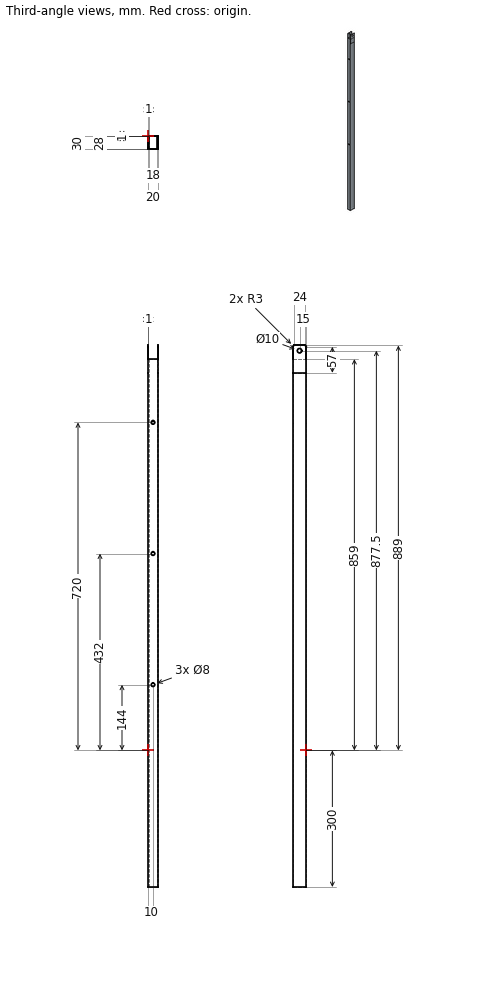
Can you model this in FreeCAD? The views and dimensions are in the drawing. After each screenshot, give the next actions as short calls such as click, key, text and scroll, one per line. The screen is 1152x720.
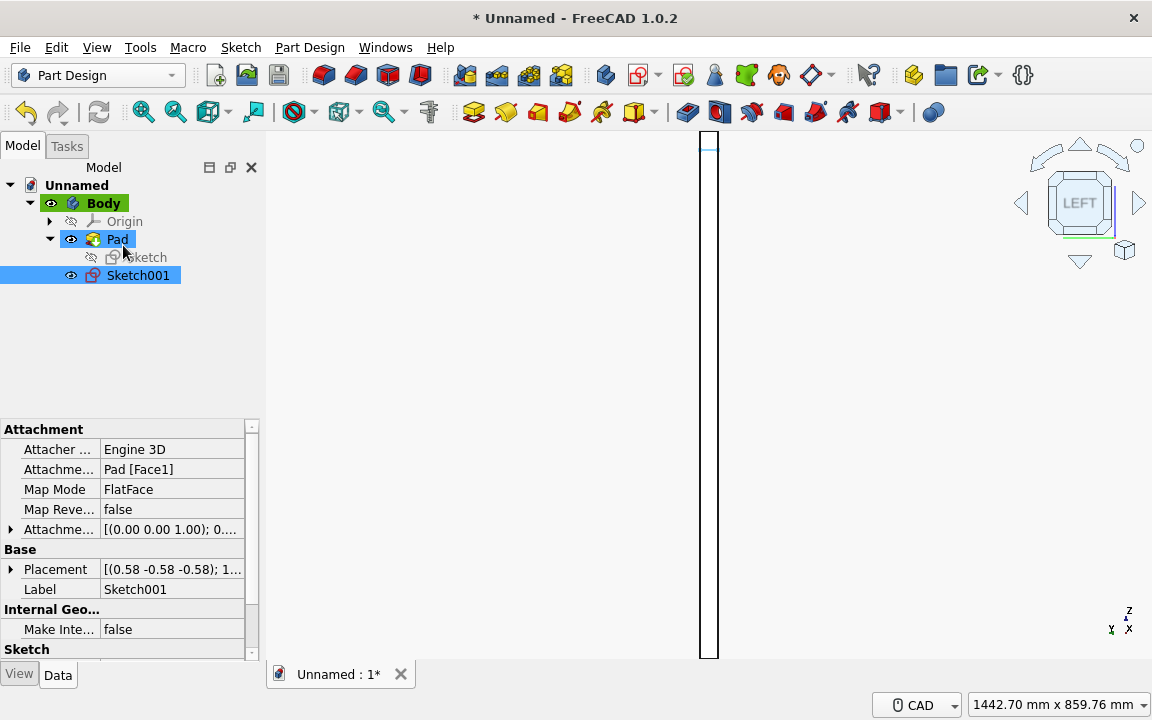
click(474, 112)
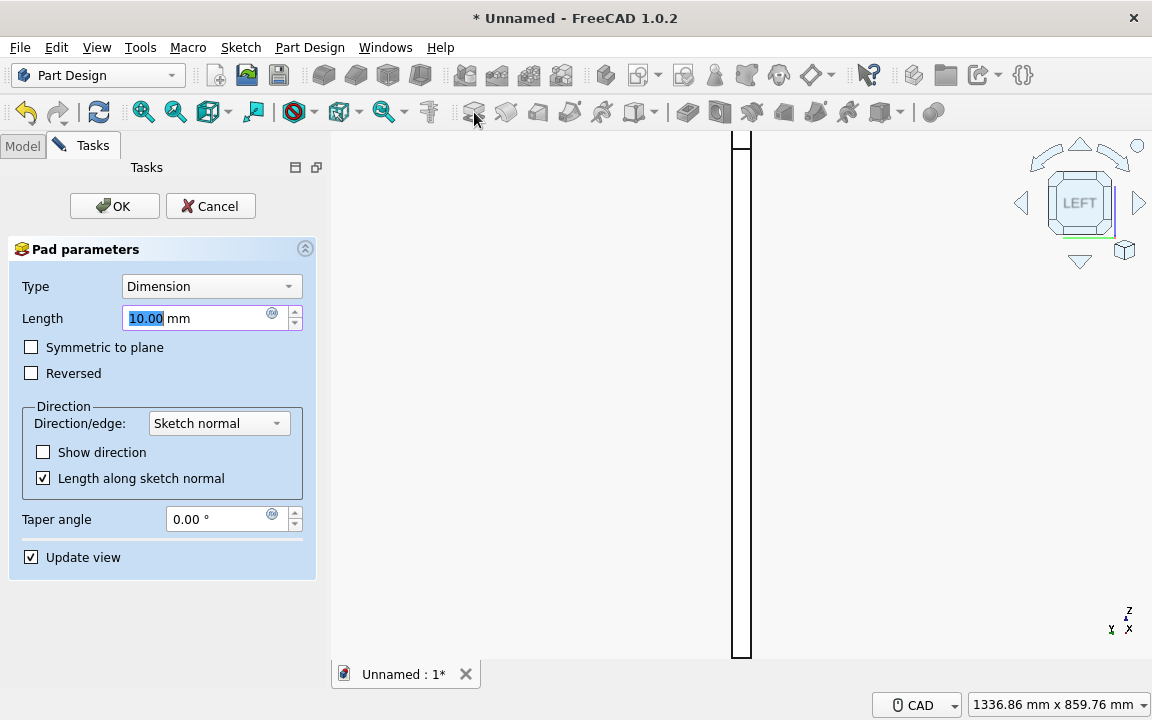
text(1)
key(Tab)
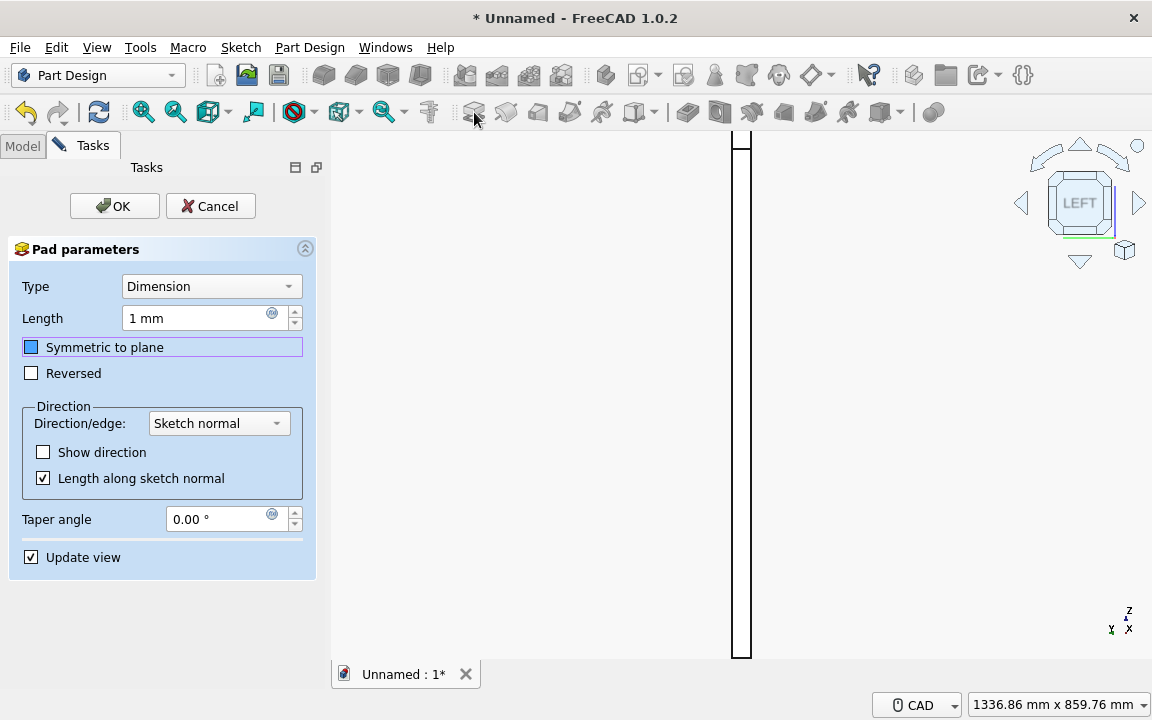
click(115, 206)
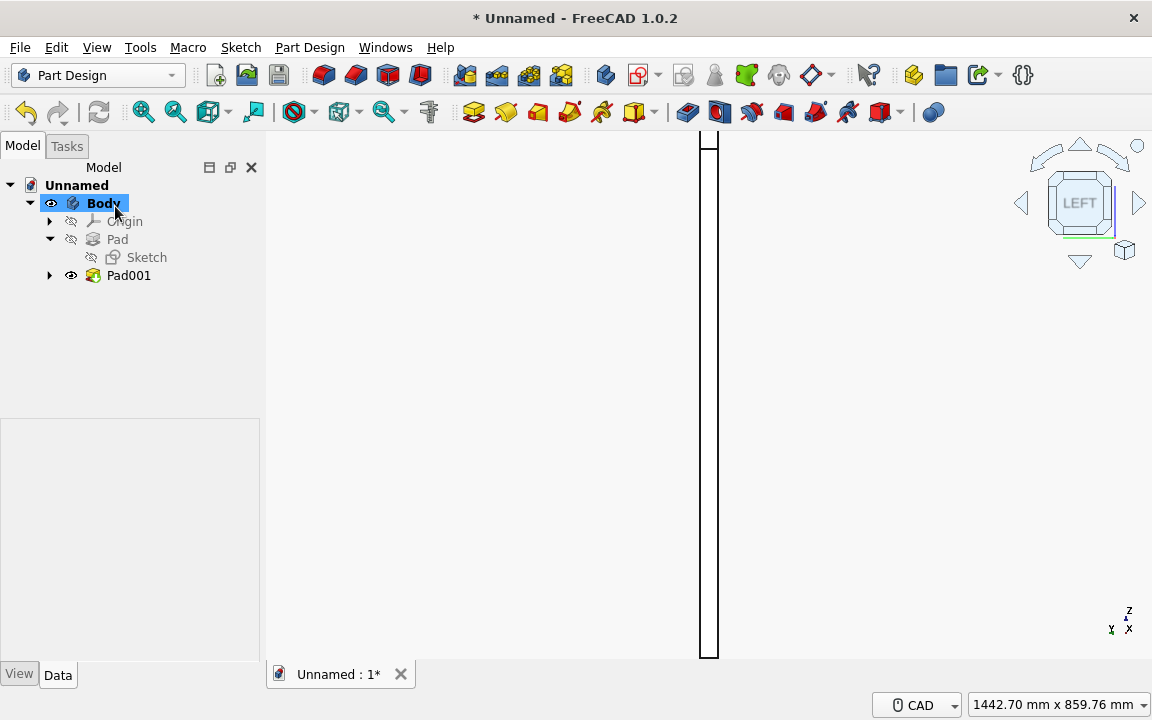
key(v)
key(f)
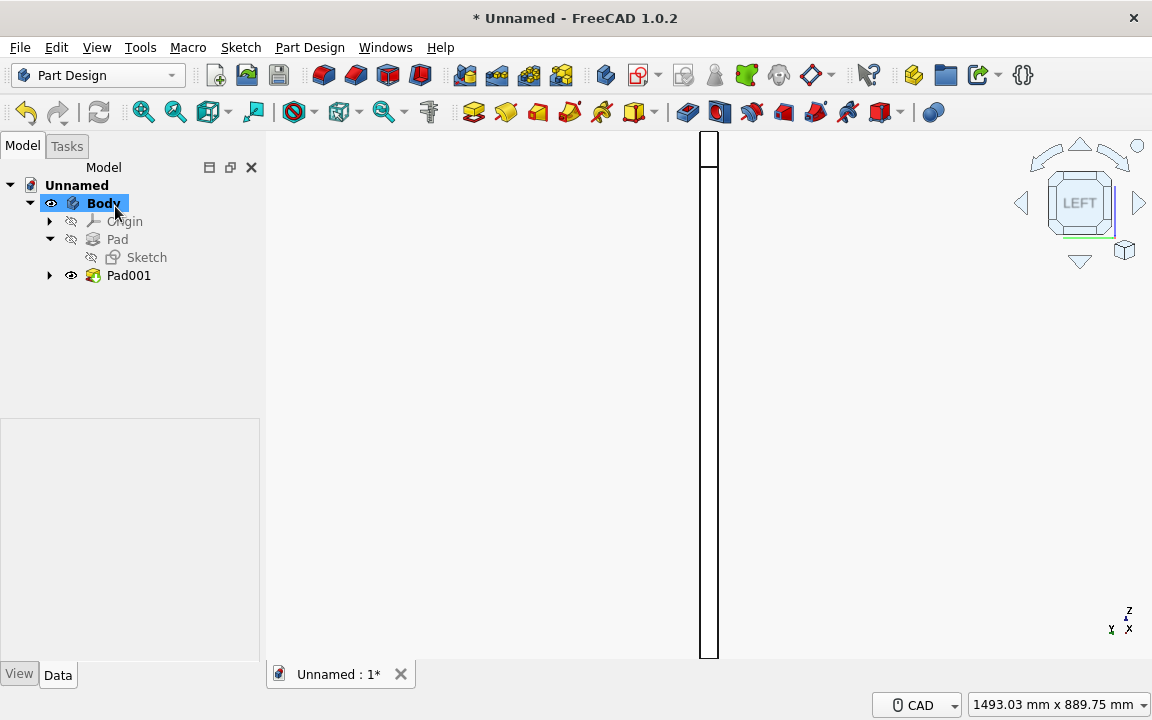
click(50, 221)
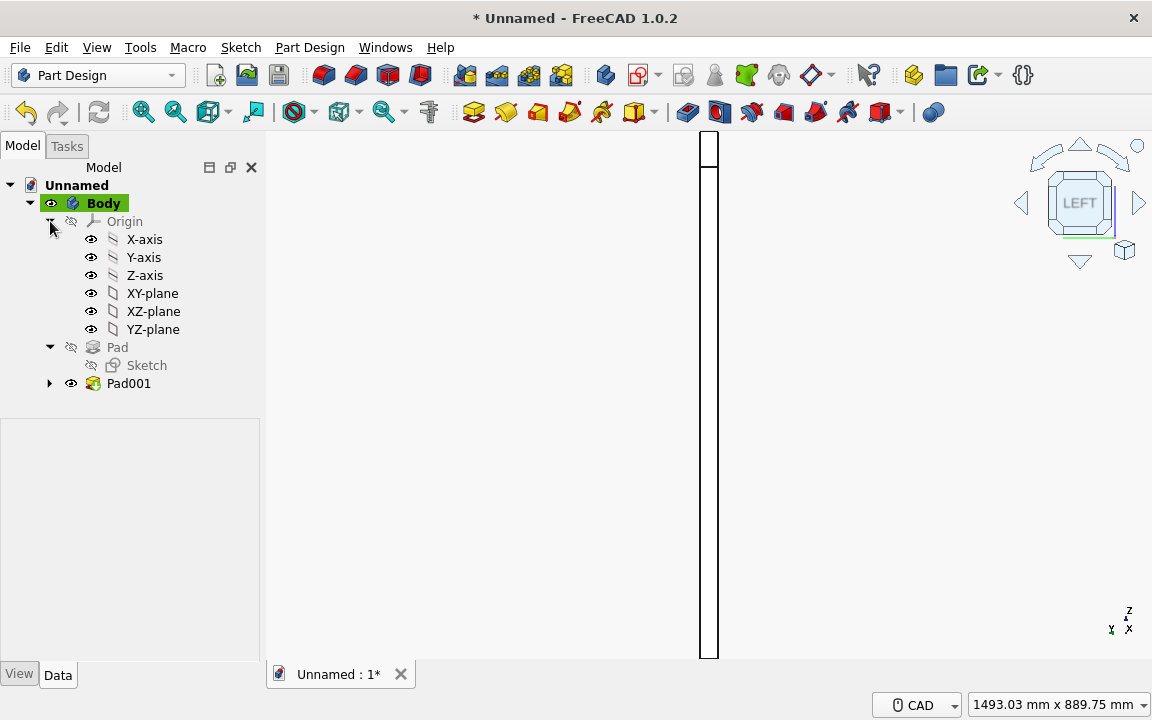
click(136, 329)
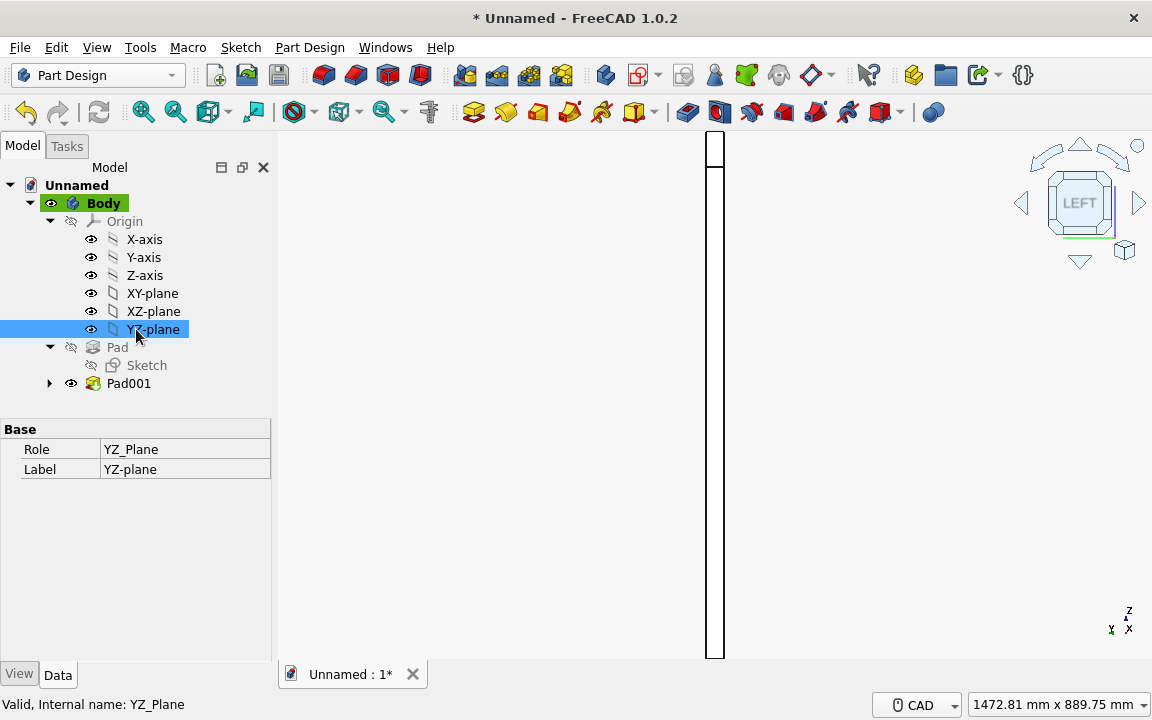
click(812, 76)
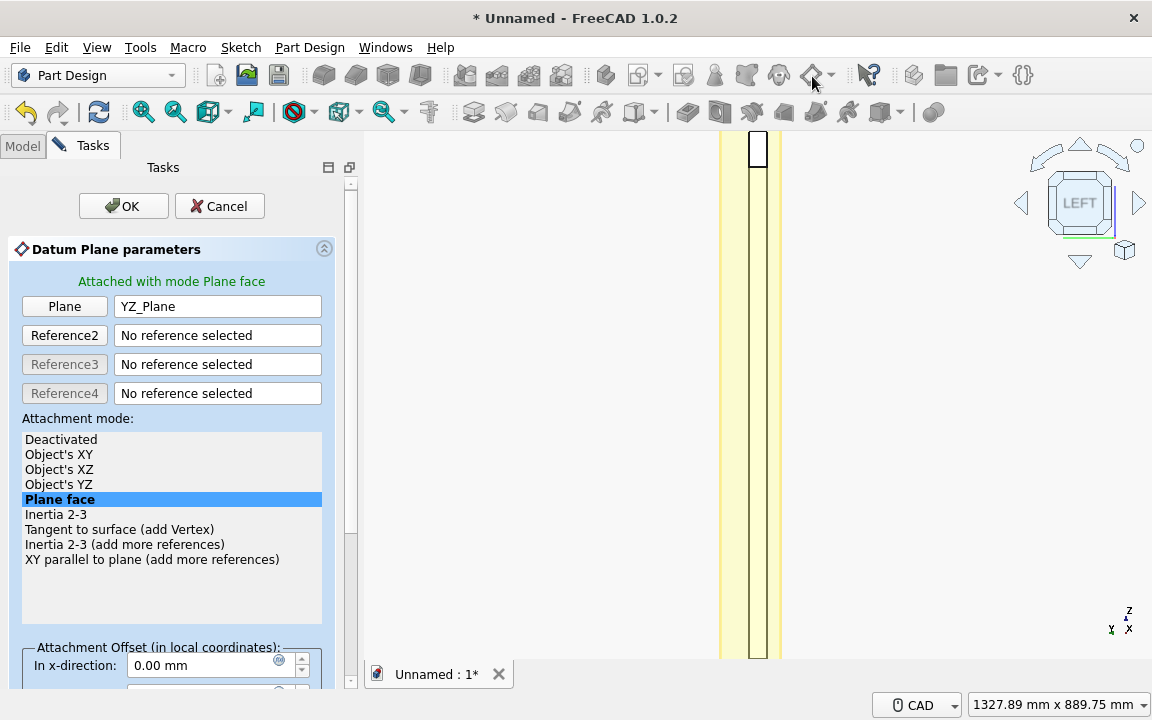
scroll(351, 432, down, 2)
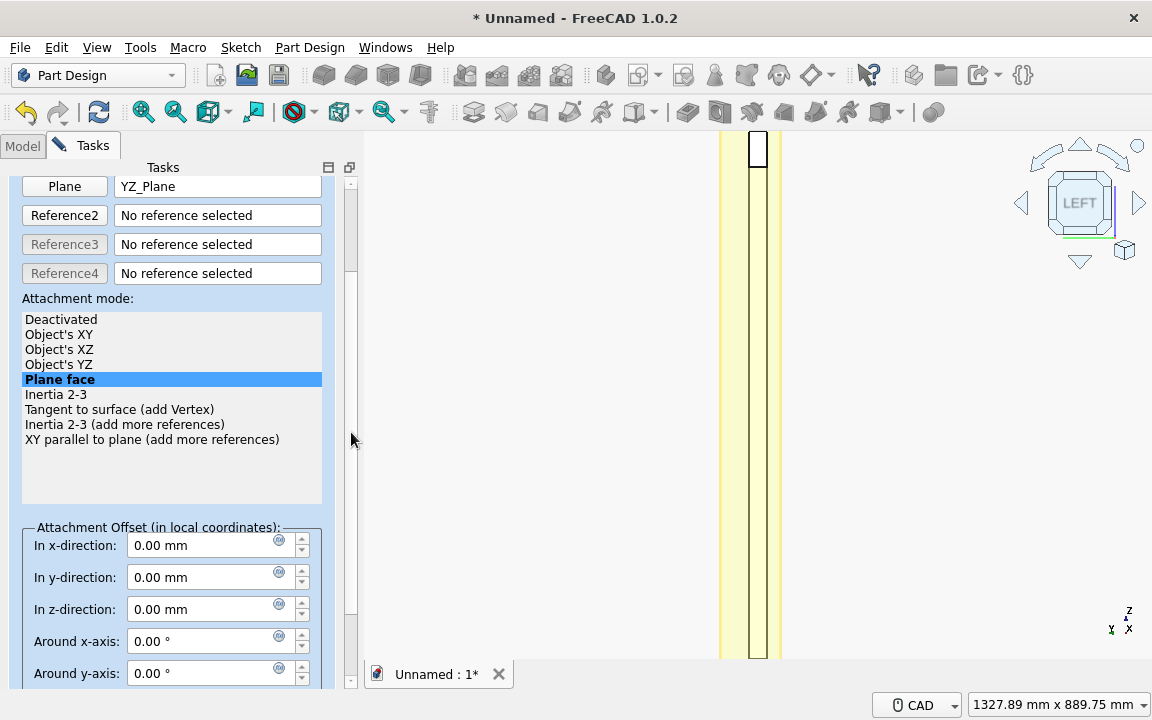
triple_click(210, 609)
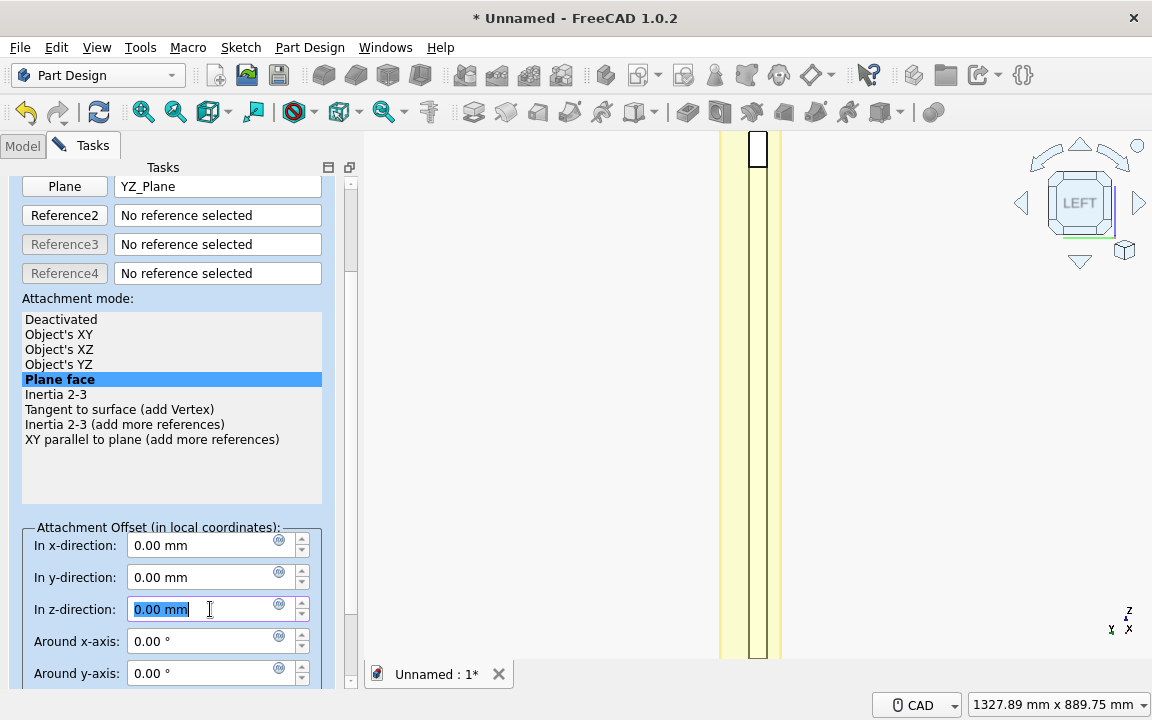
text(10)
key(Tab)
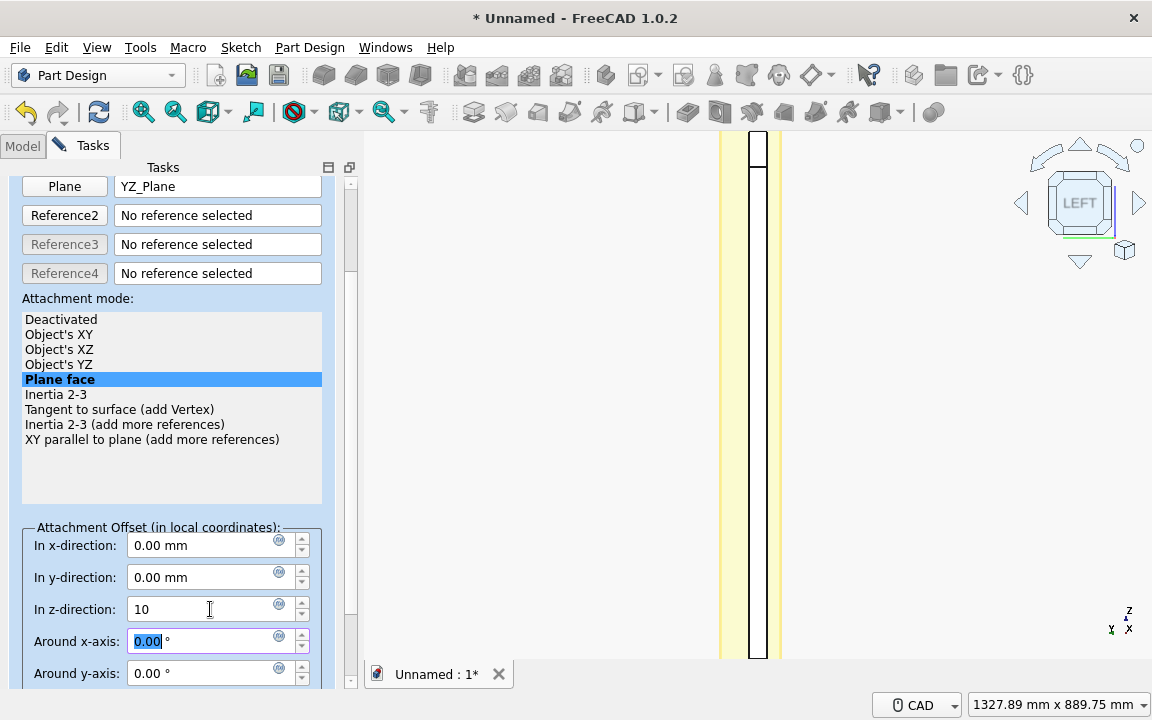
scroll(351, 432, up, 3)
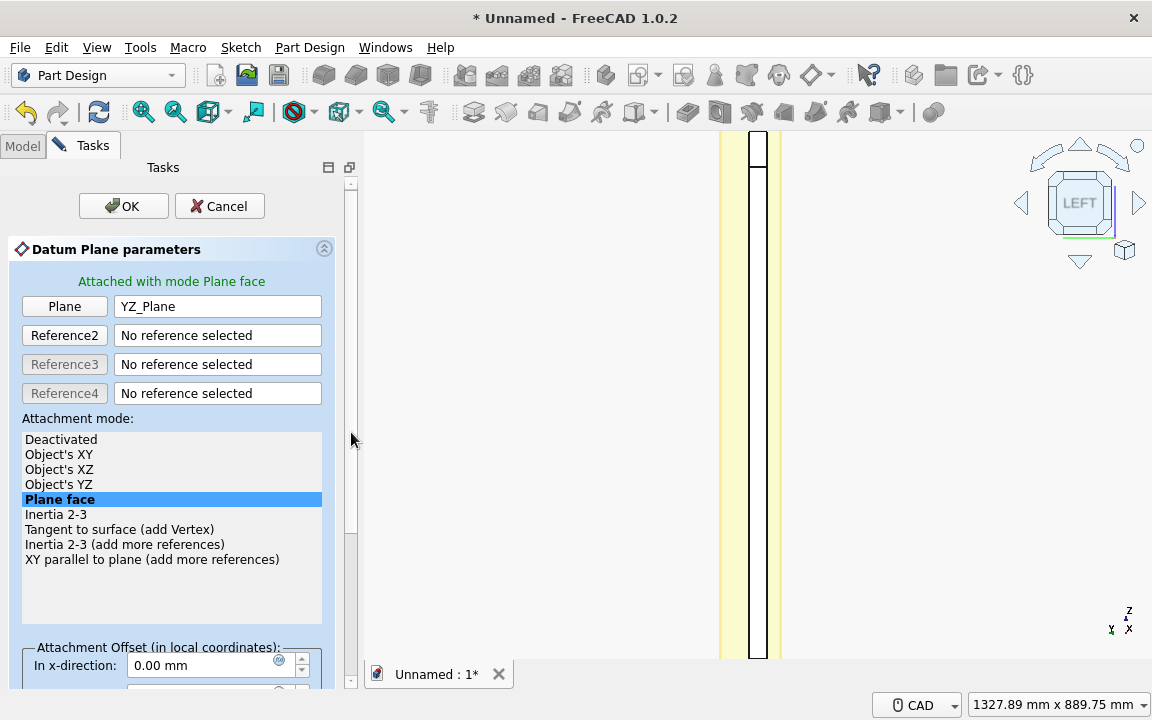
click(124, 206)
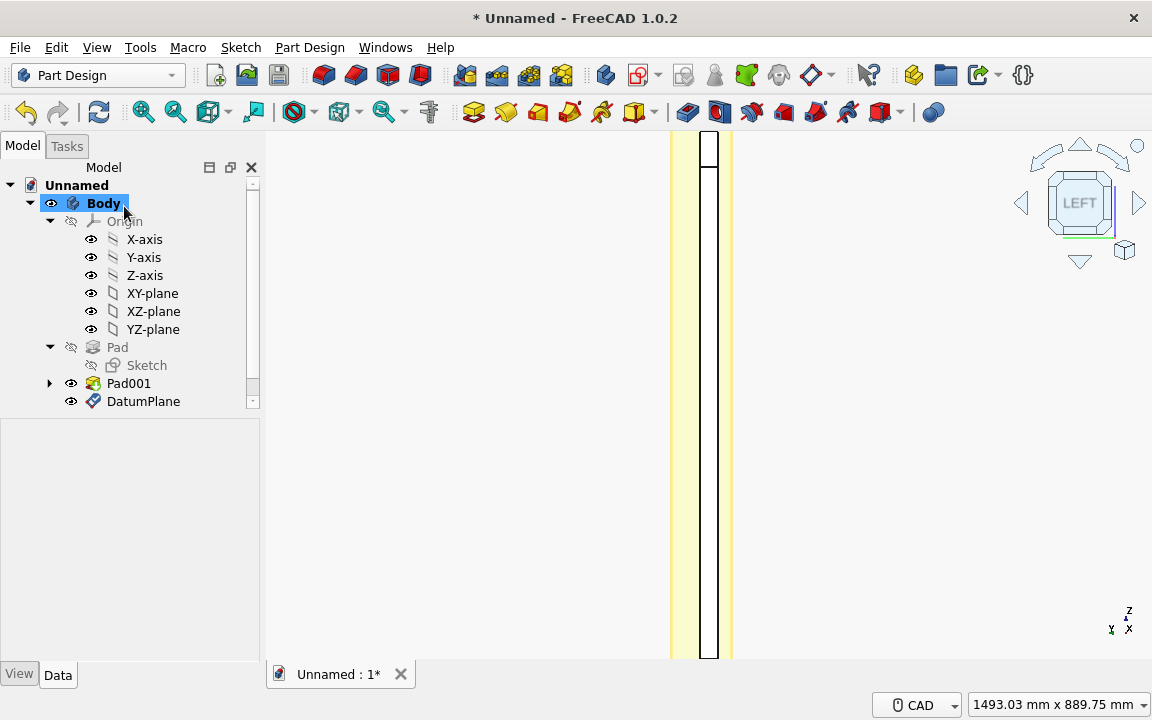
click(116, 383)